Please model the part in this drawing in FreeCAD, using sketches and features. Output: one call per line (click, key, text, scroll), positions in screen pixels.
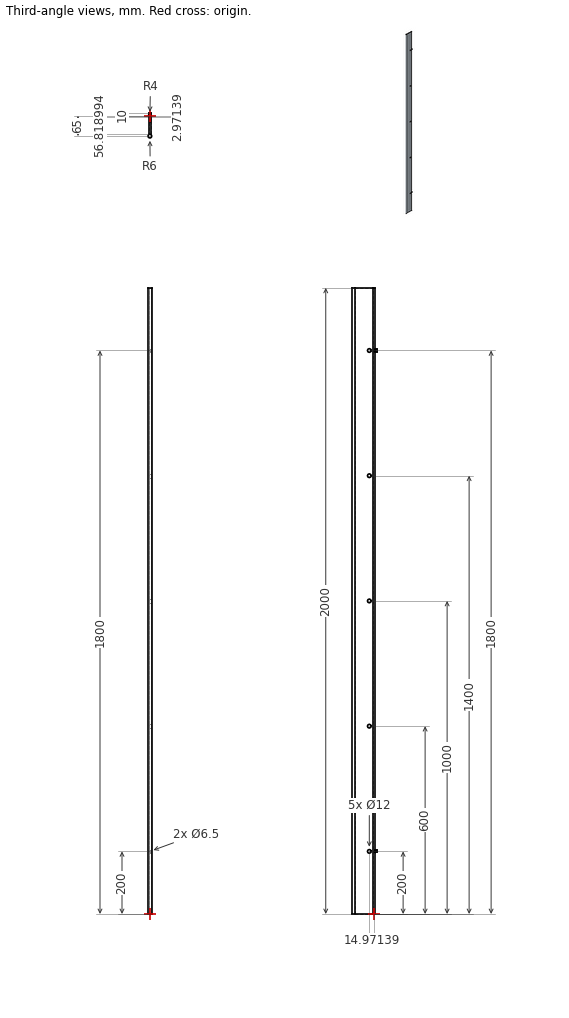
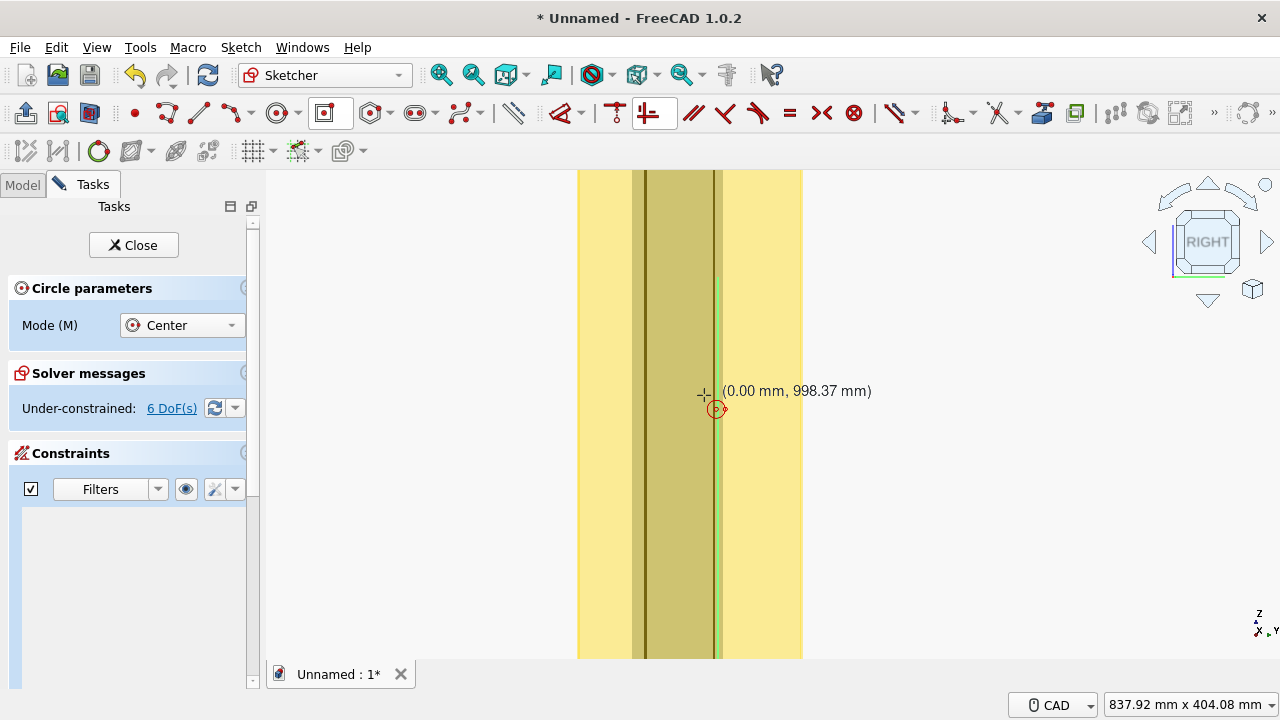
click(700, 394)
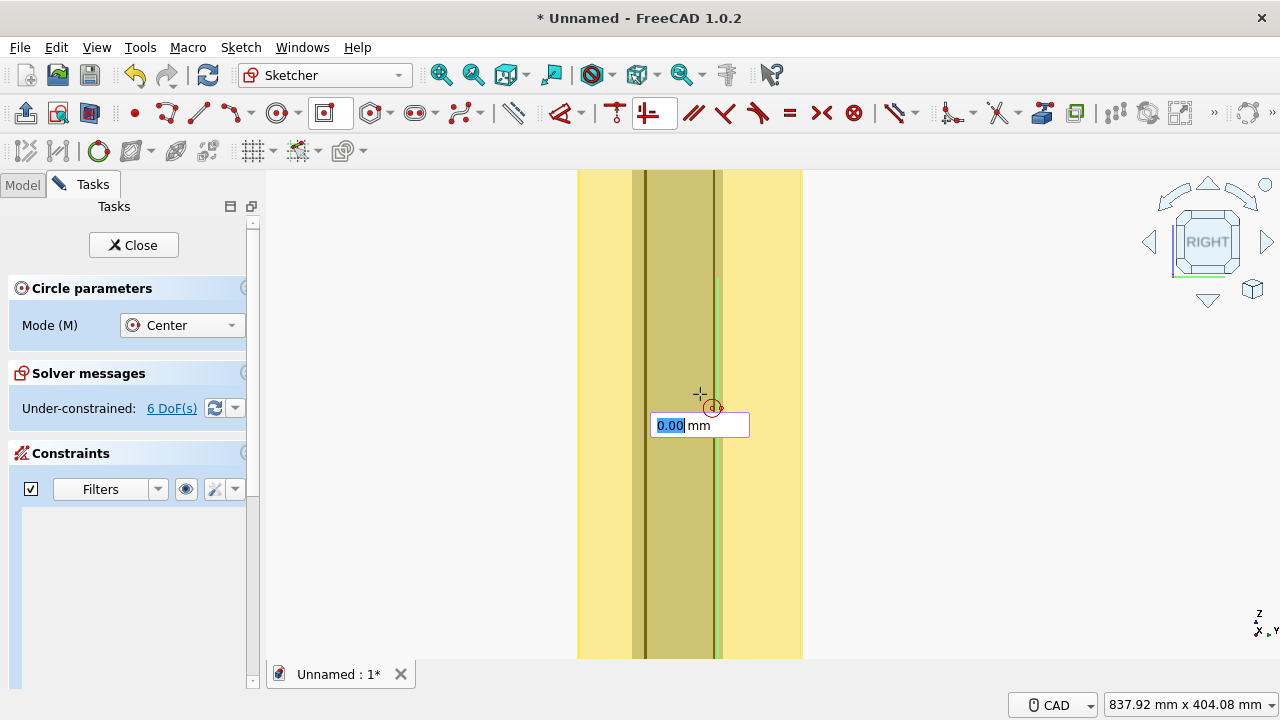
scroll(694, 389, up, 4)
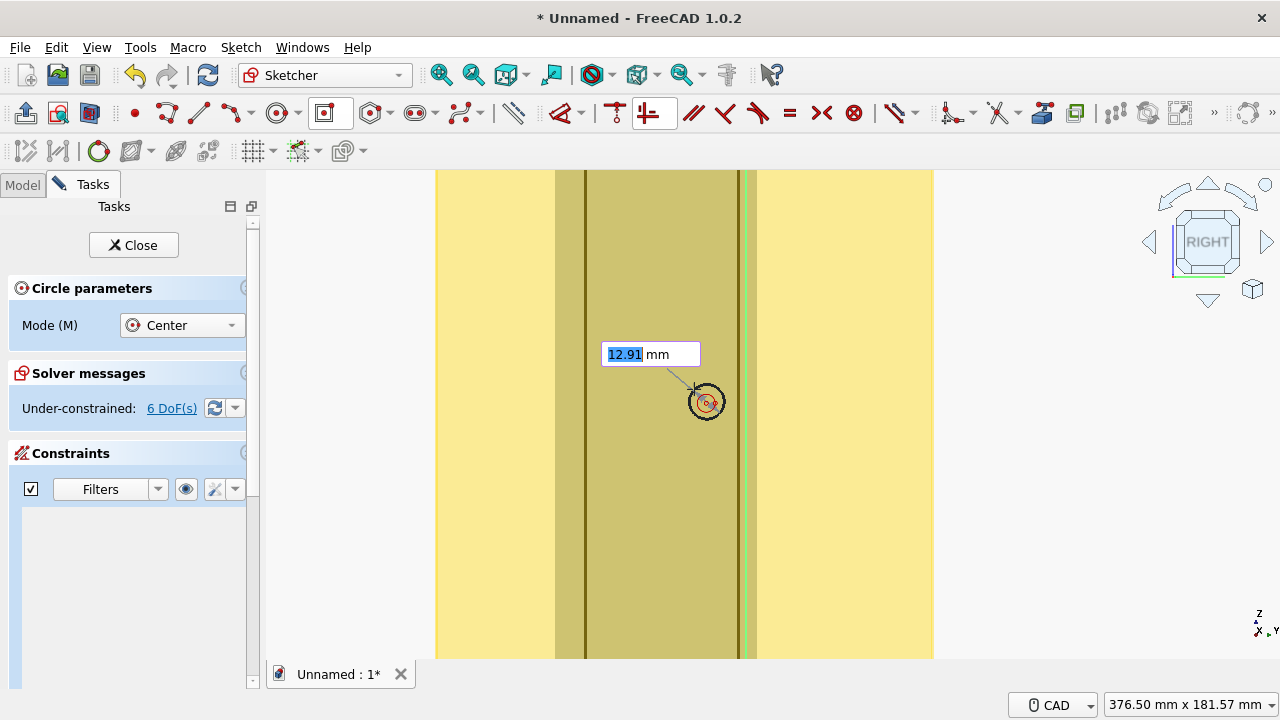
click(694, 387)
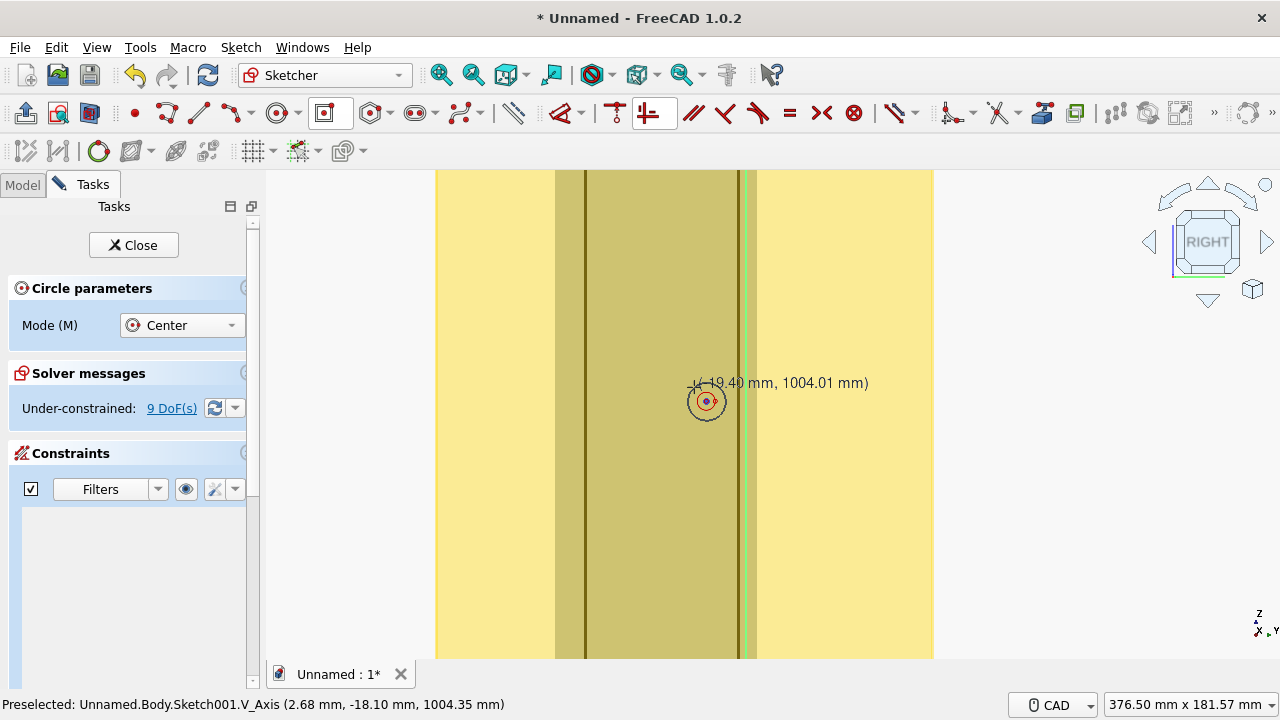
scroll(704, 399, down, 14)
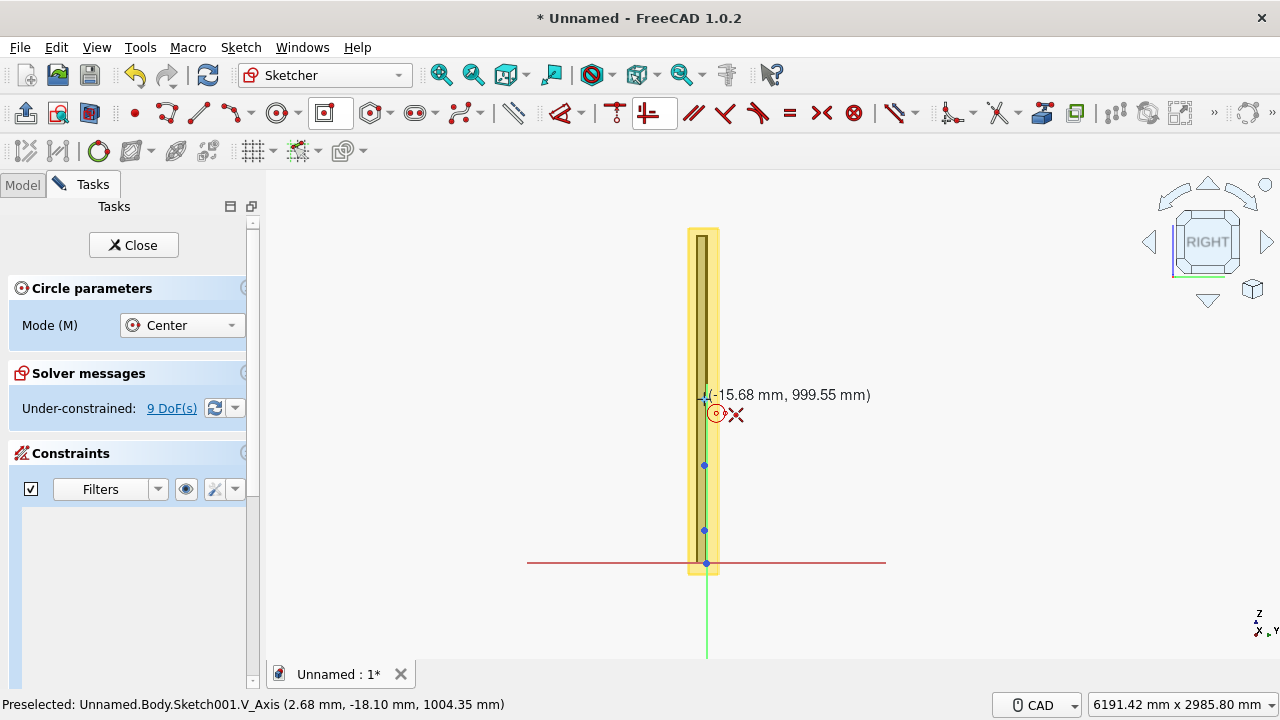
scroll(705, 334, up, 16)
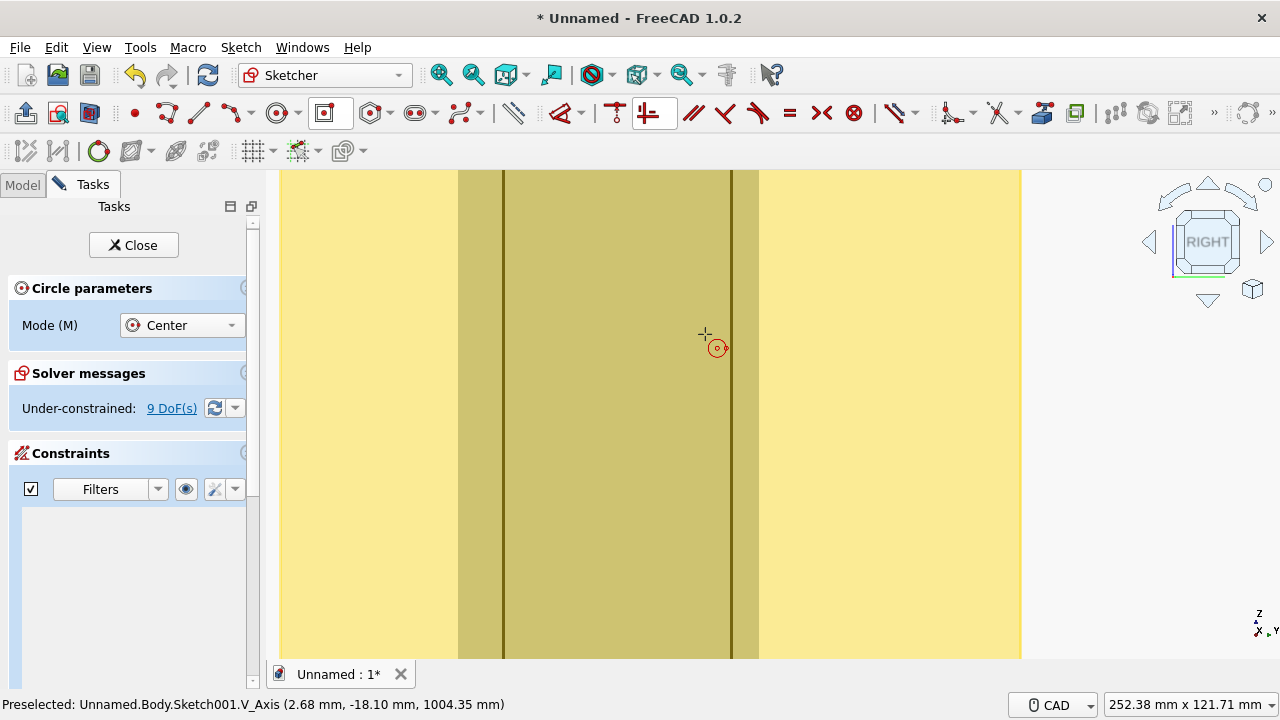
scroll(705, 315, down, 15)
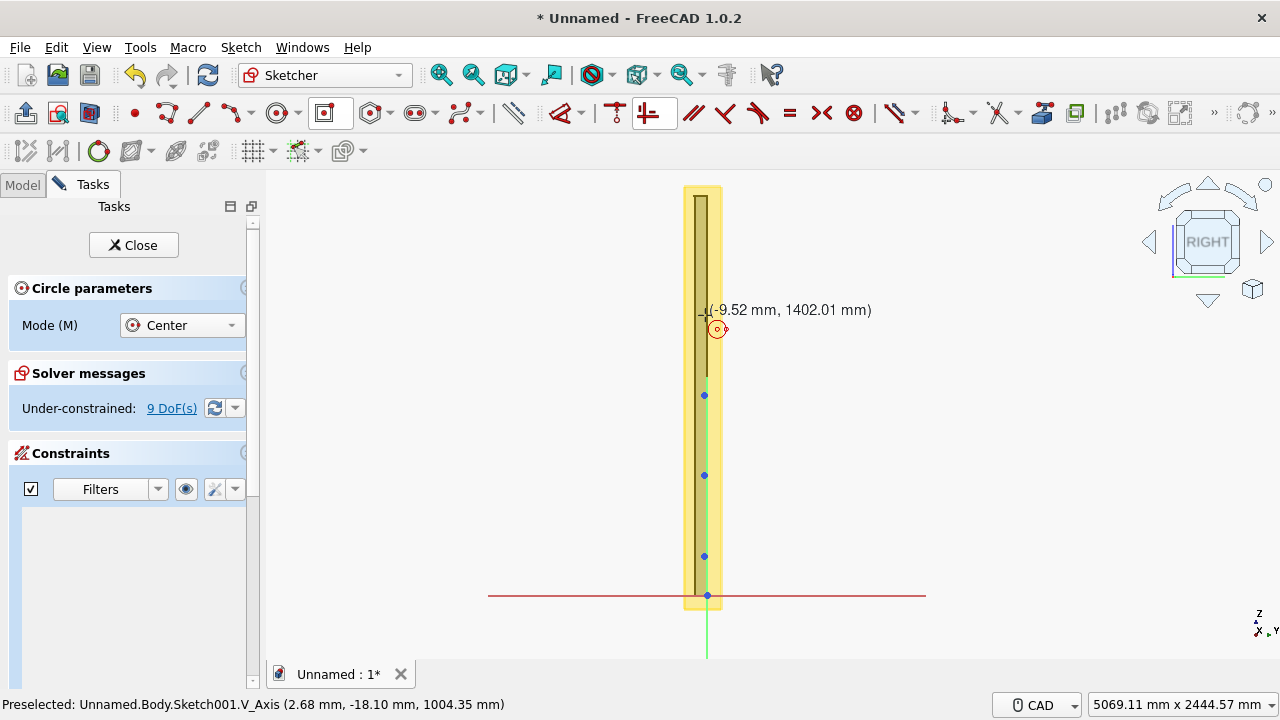
scroll(704, 316, up, 9)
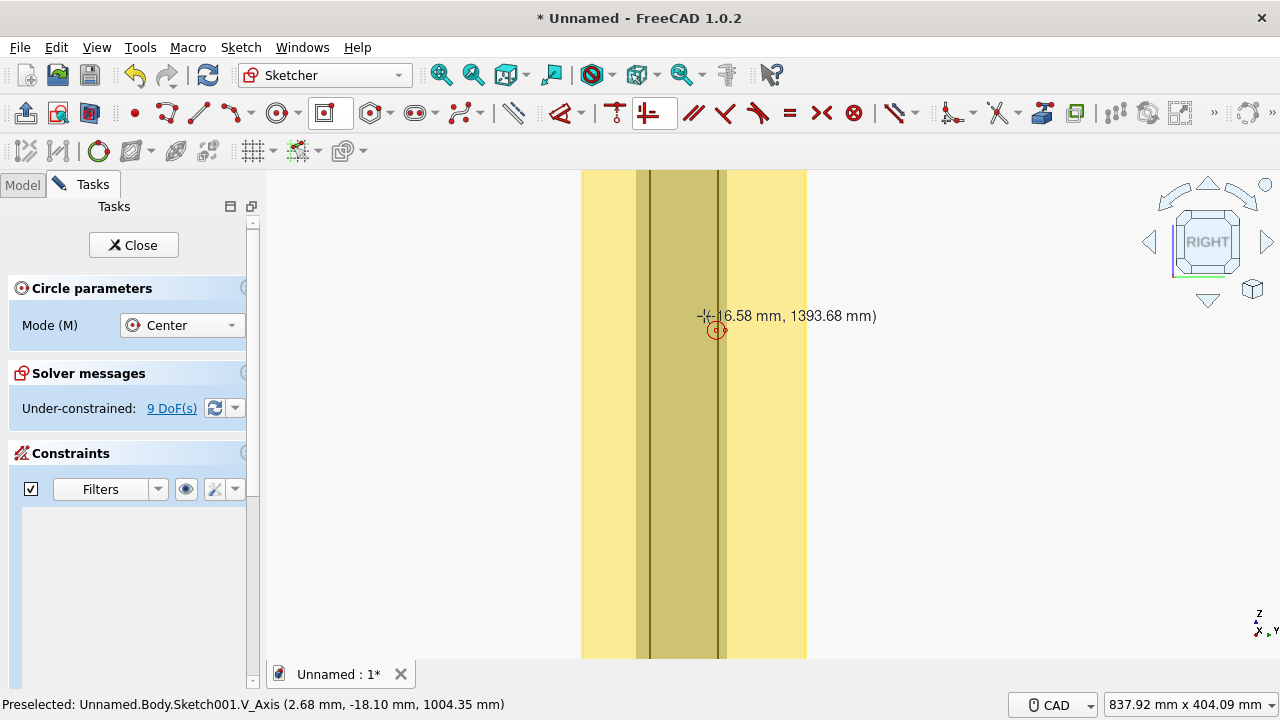
click(704, 313)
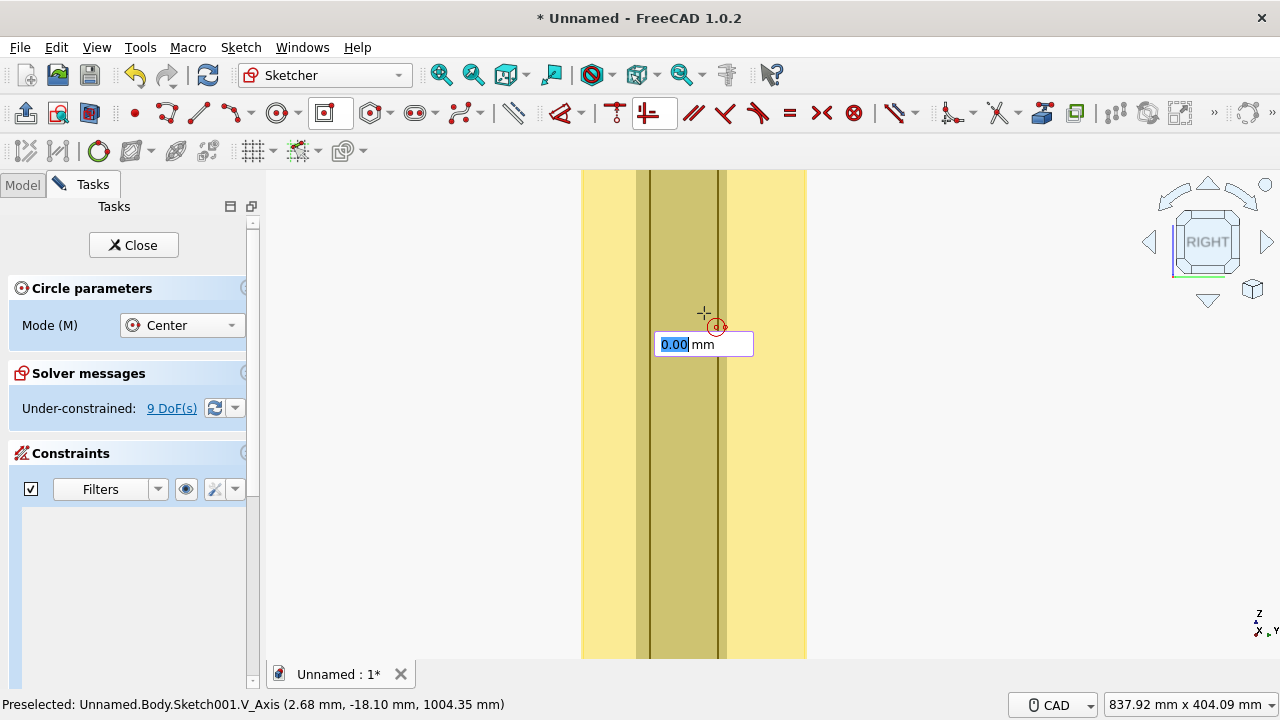
scroll(699, 308, up, 4)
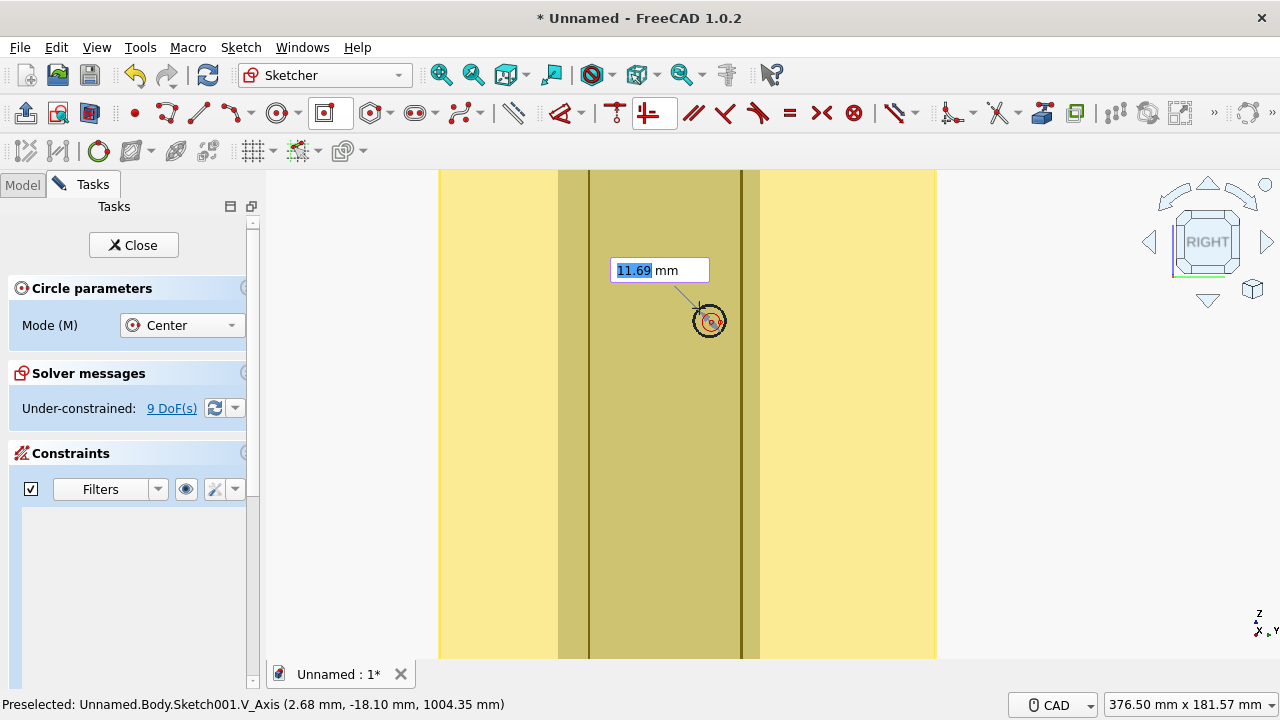
click(698, 307)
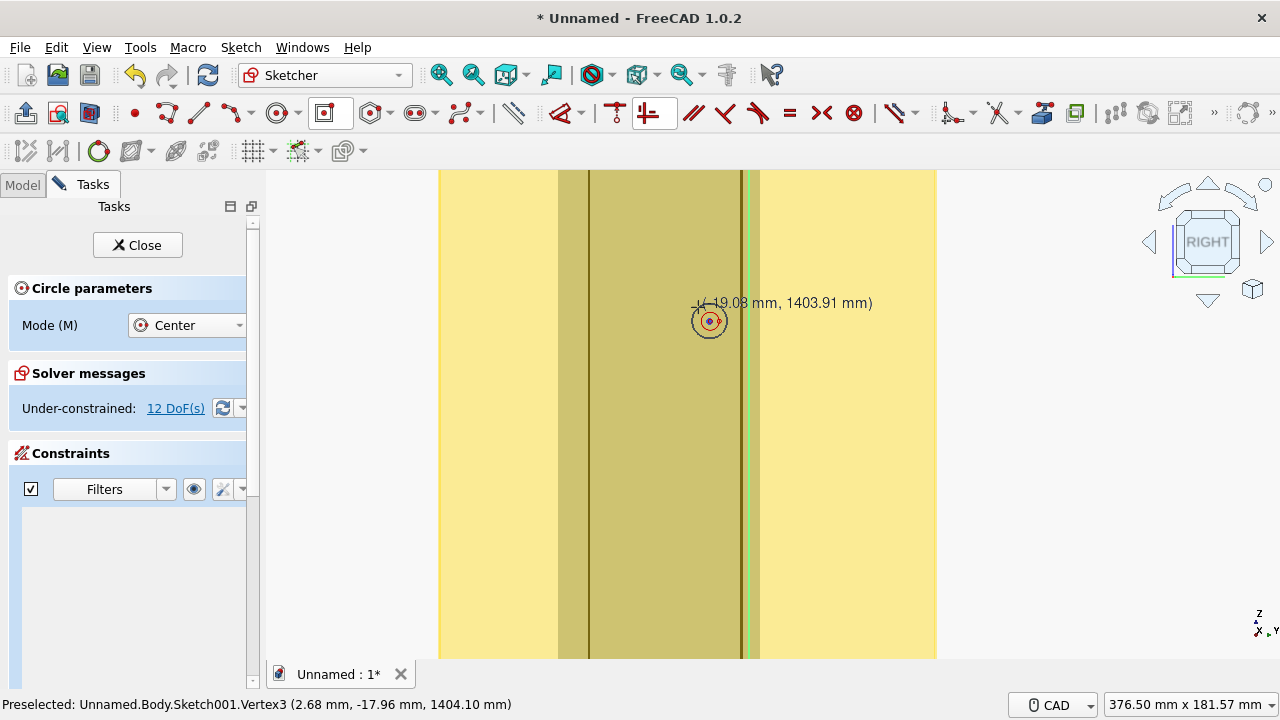
scroll(703, 334, down, 14)